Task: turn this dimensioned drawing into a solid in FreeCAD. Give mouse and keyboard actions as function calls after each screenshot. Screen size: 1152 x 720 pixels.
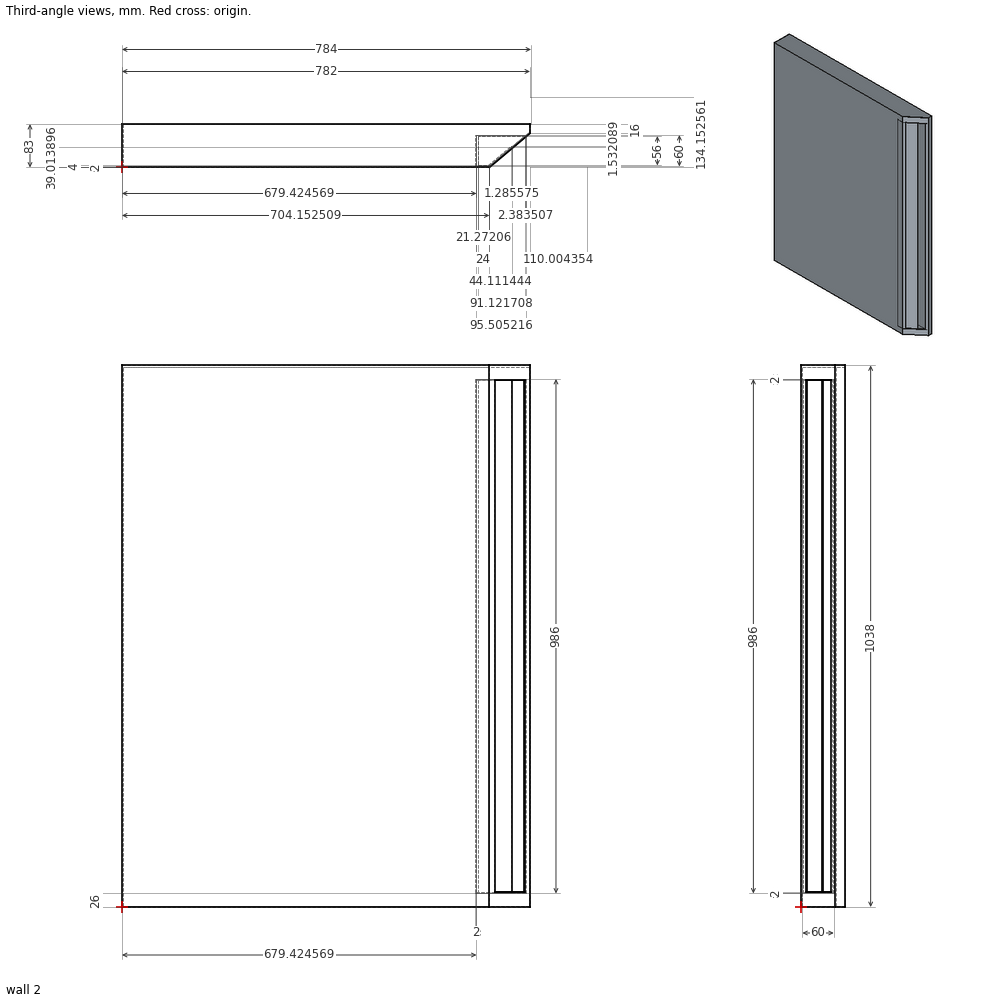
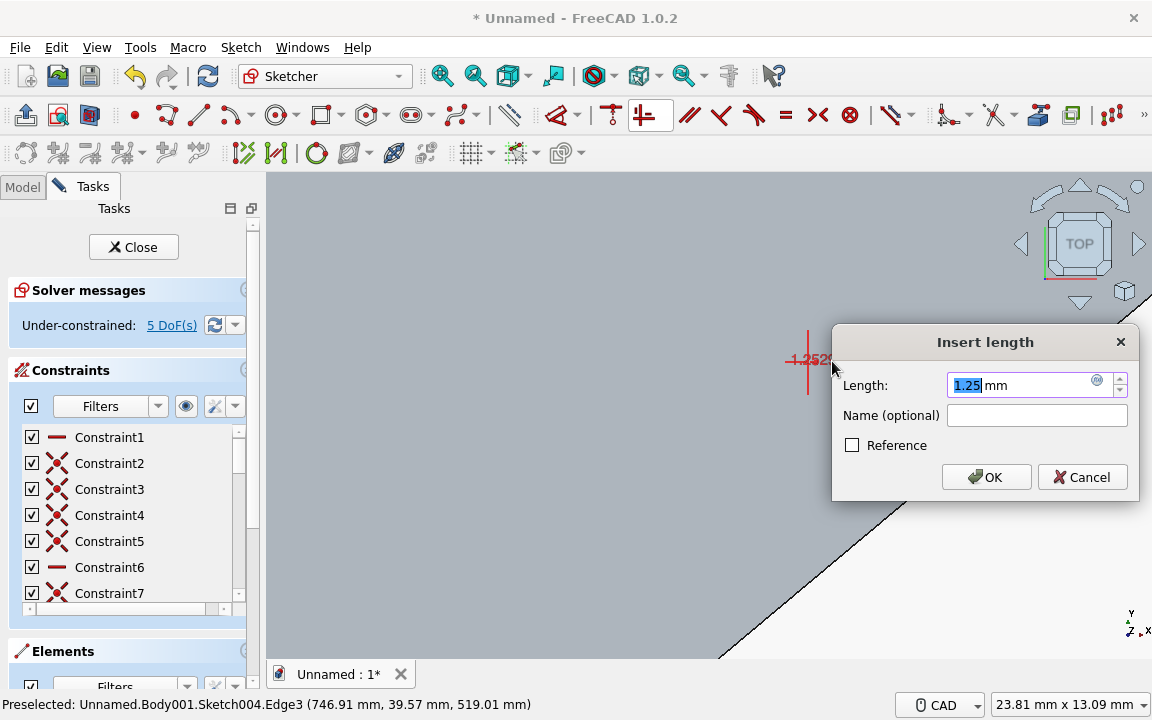
text(1.285575)
key(Return)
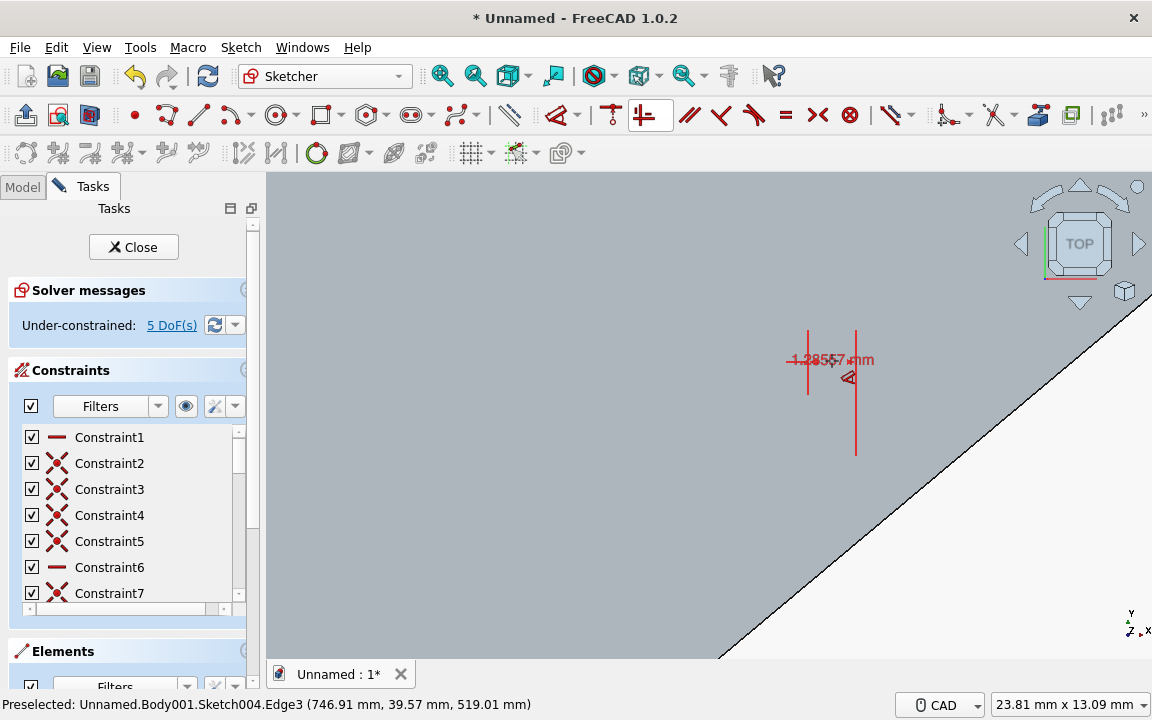
click(842, 437)
click(890, 425)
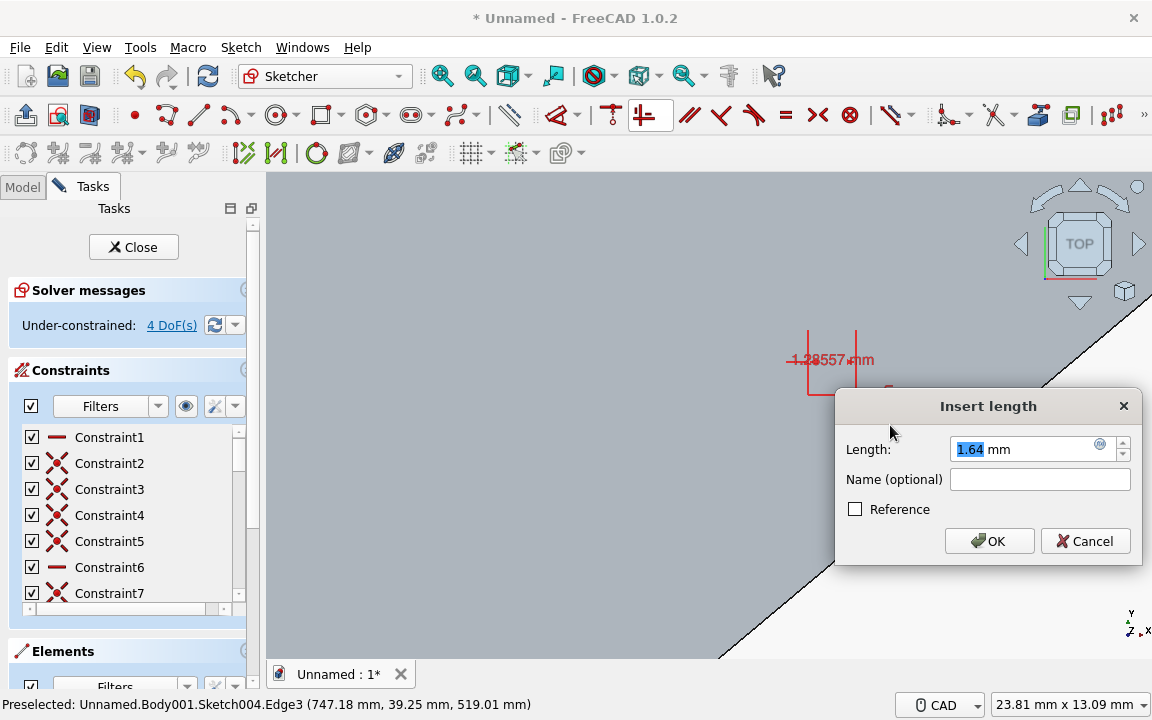
text(1.532089)
key(Return)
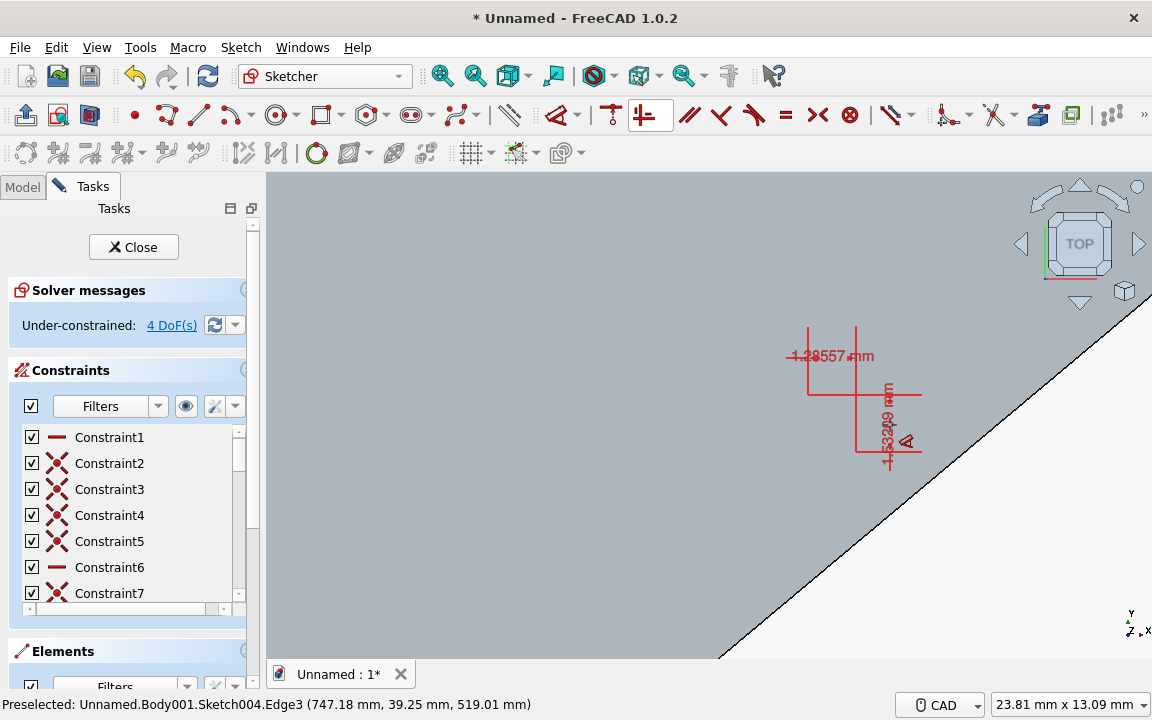
scroll(725, 370, down, 10)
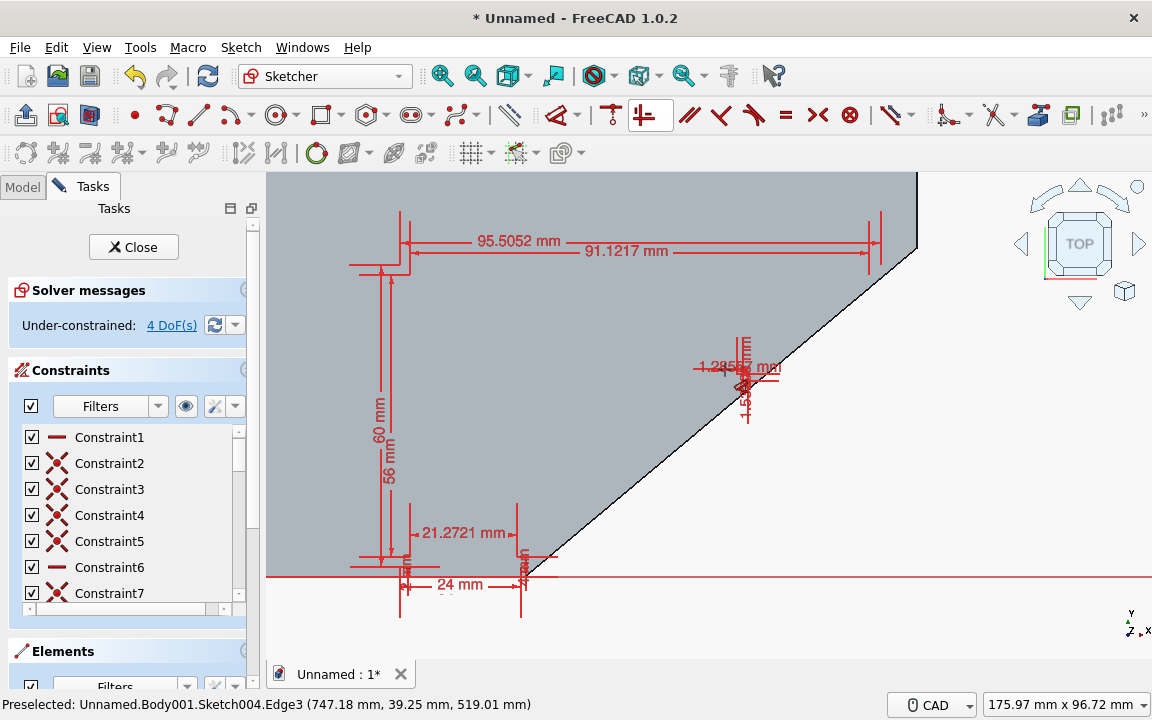
scroll(873, 272, up, 6)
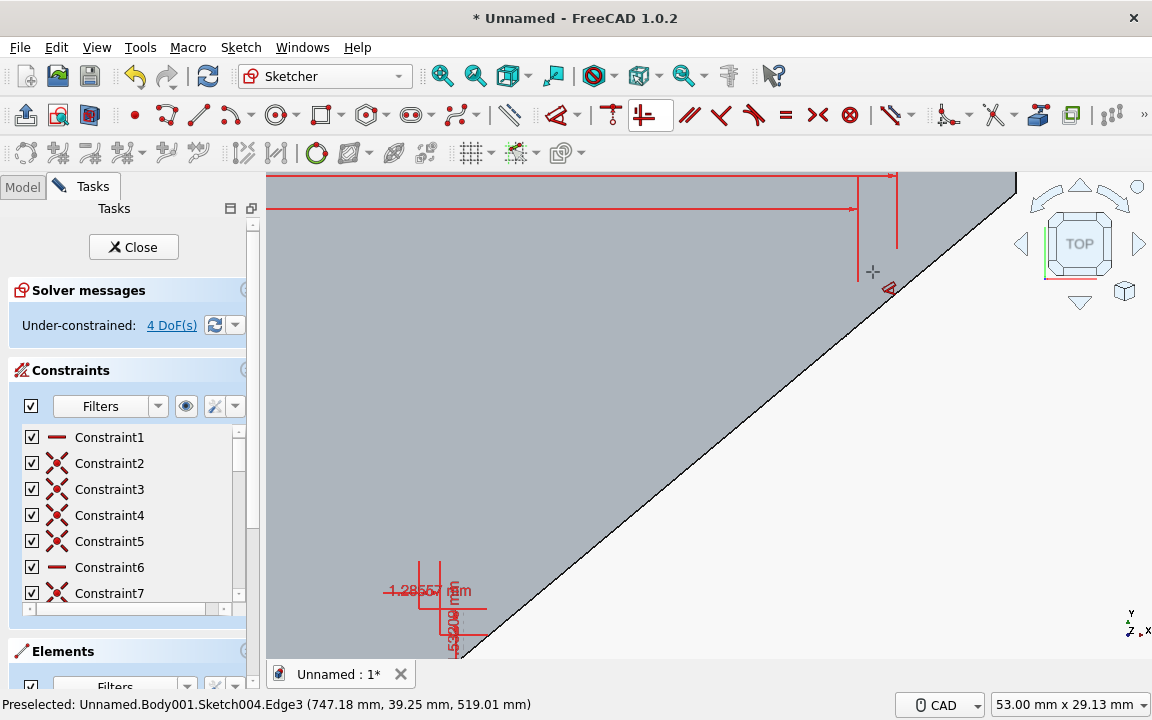
click(870, 272)
click(878, 214)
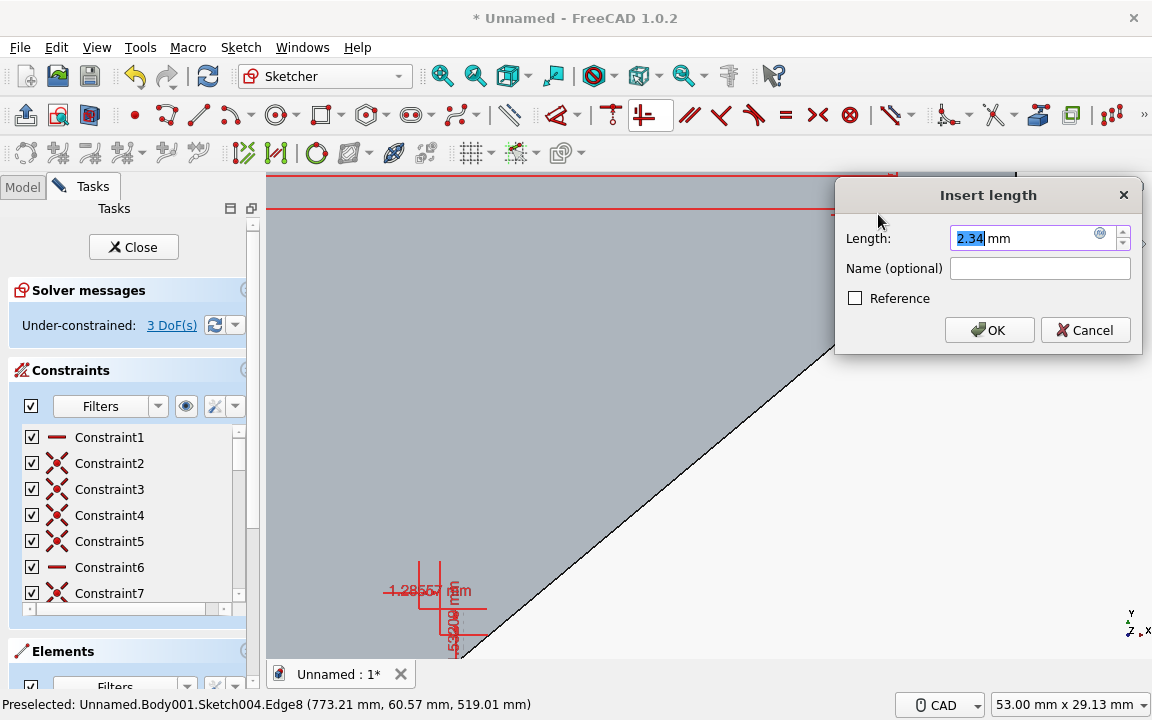
text(2.383507)
key(Return)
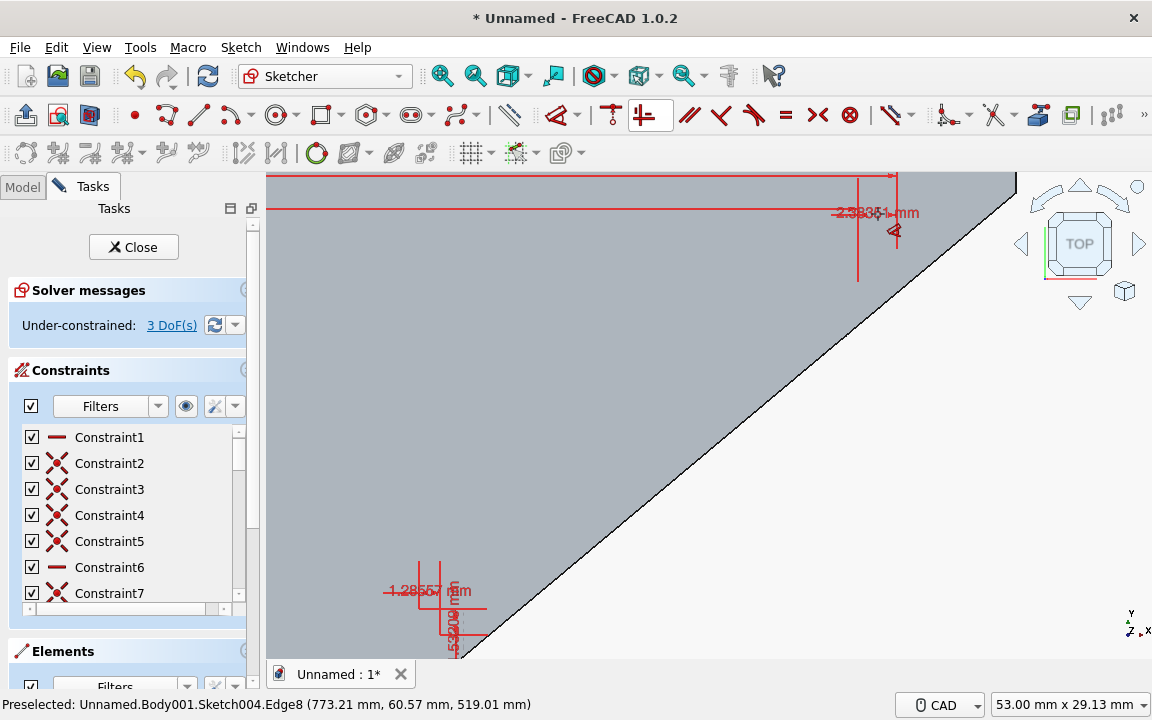
scroll(874, 271, down, 6)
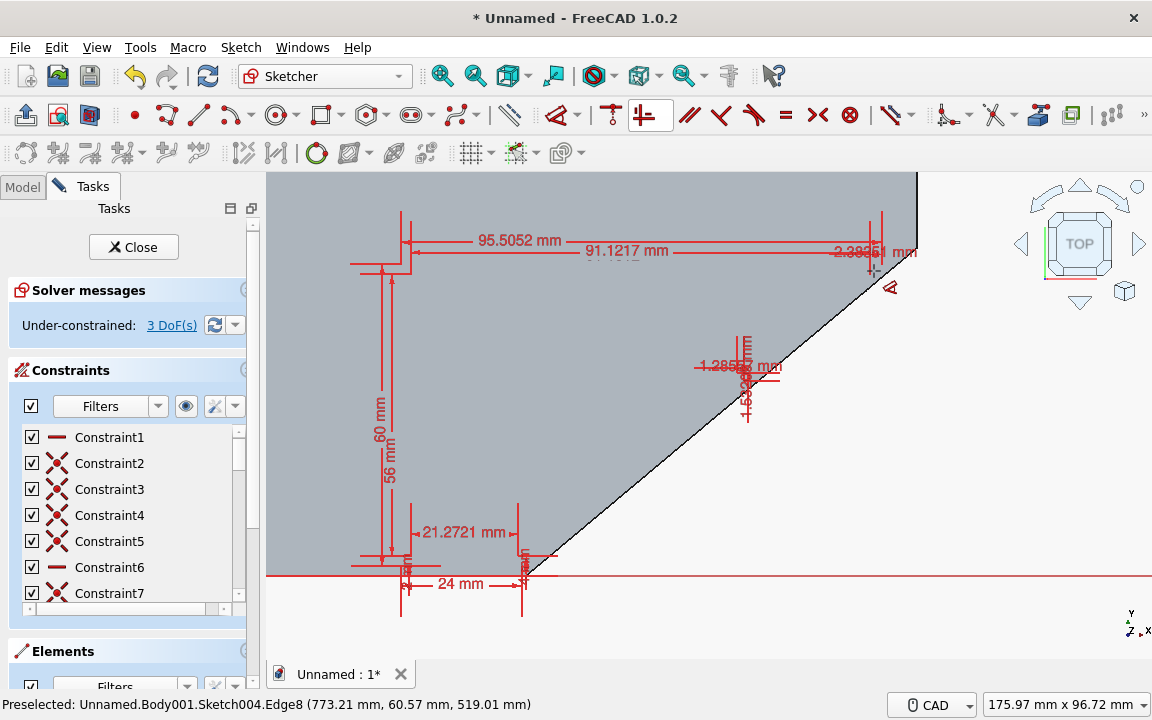
click(744, 381)
click(778, 479)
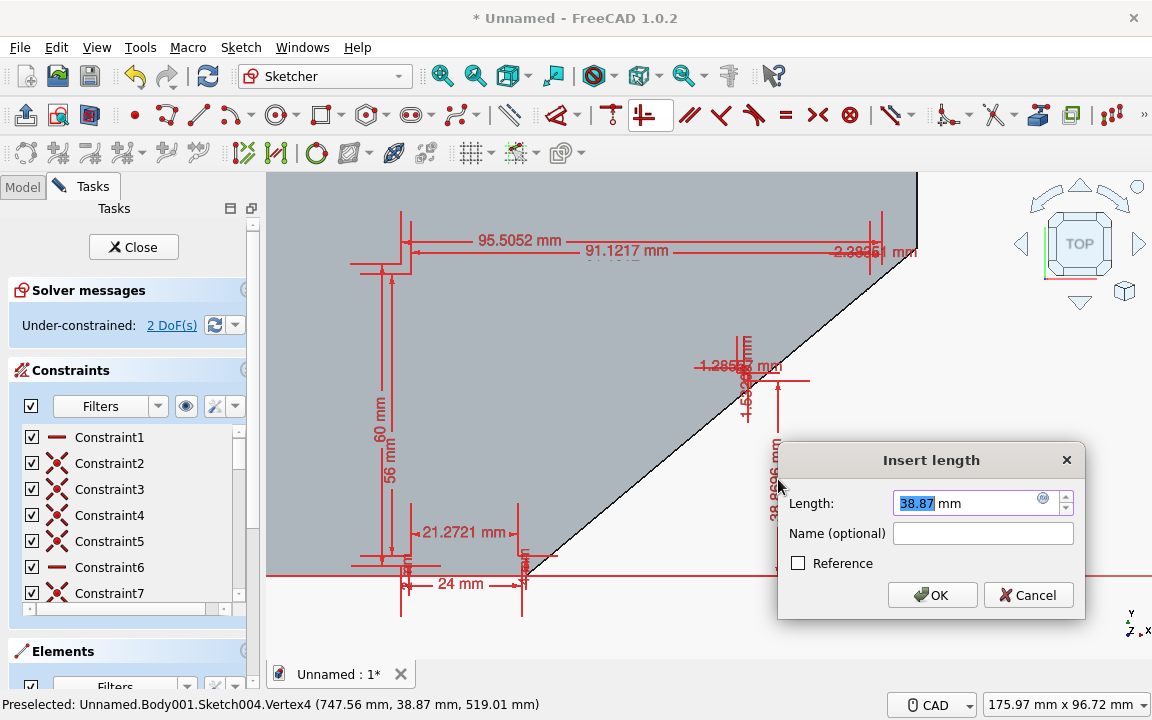
text(39.013896)
key(Return)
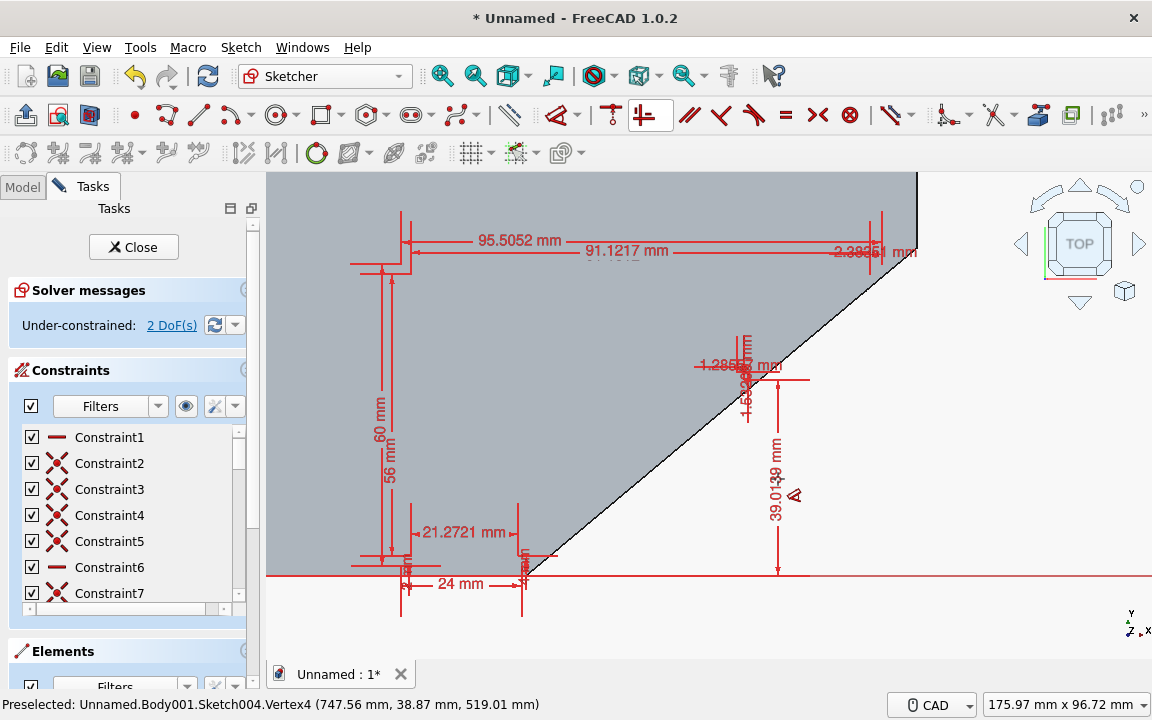
scroll(588, 510, up, 2)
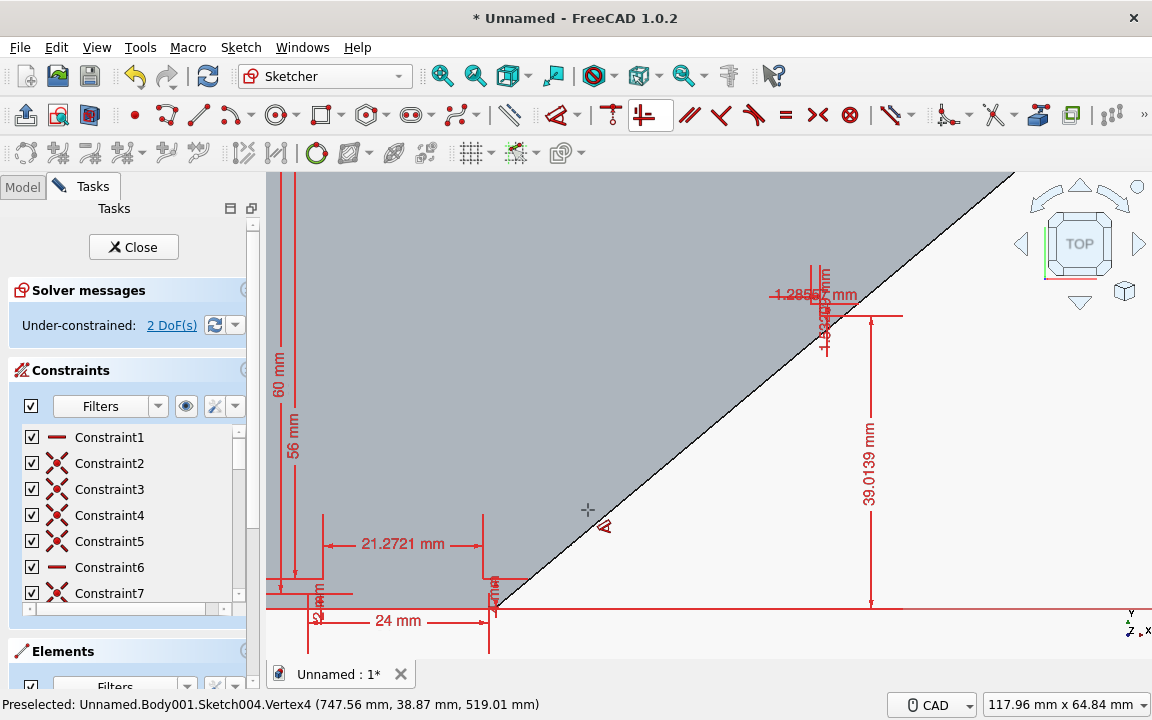
click(588, 510)
click(655, 628)